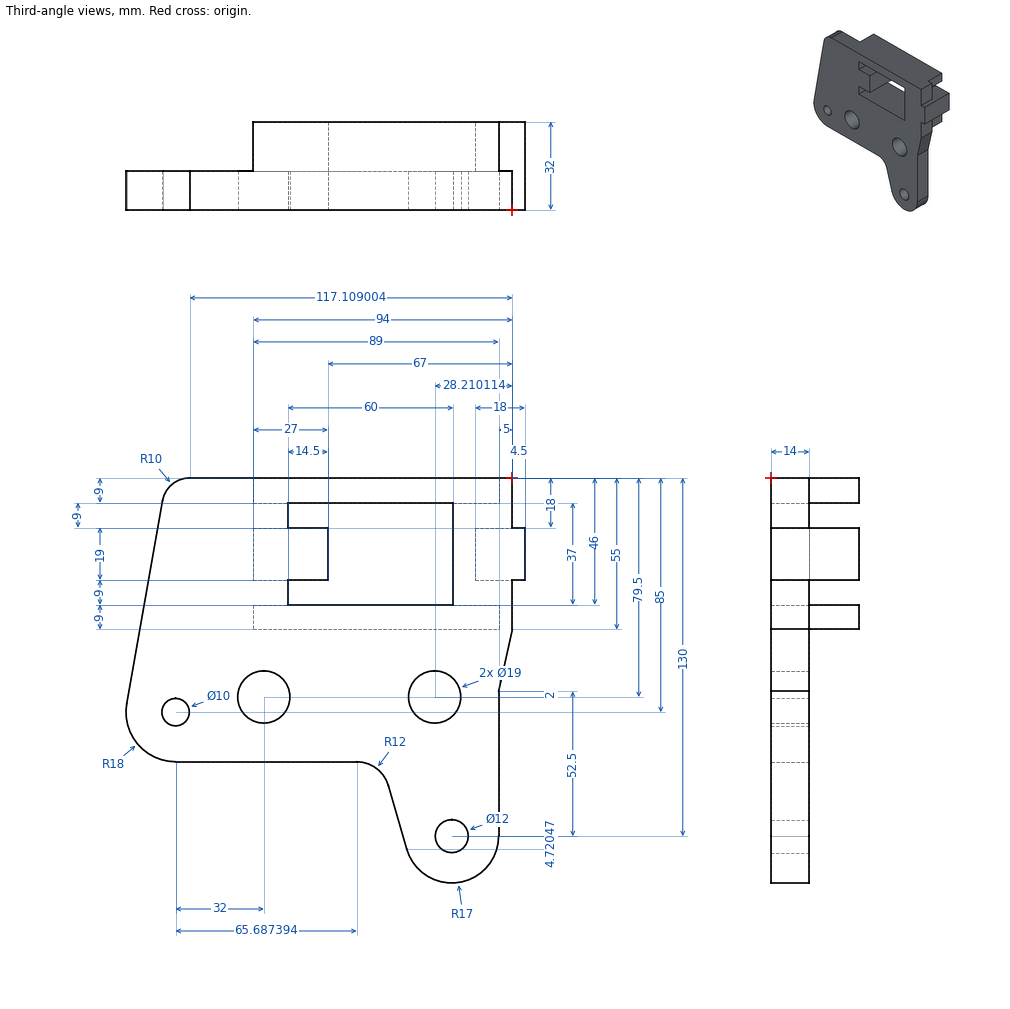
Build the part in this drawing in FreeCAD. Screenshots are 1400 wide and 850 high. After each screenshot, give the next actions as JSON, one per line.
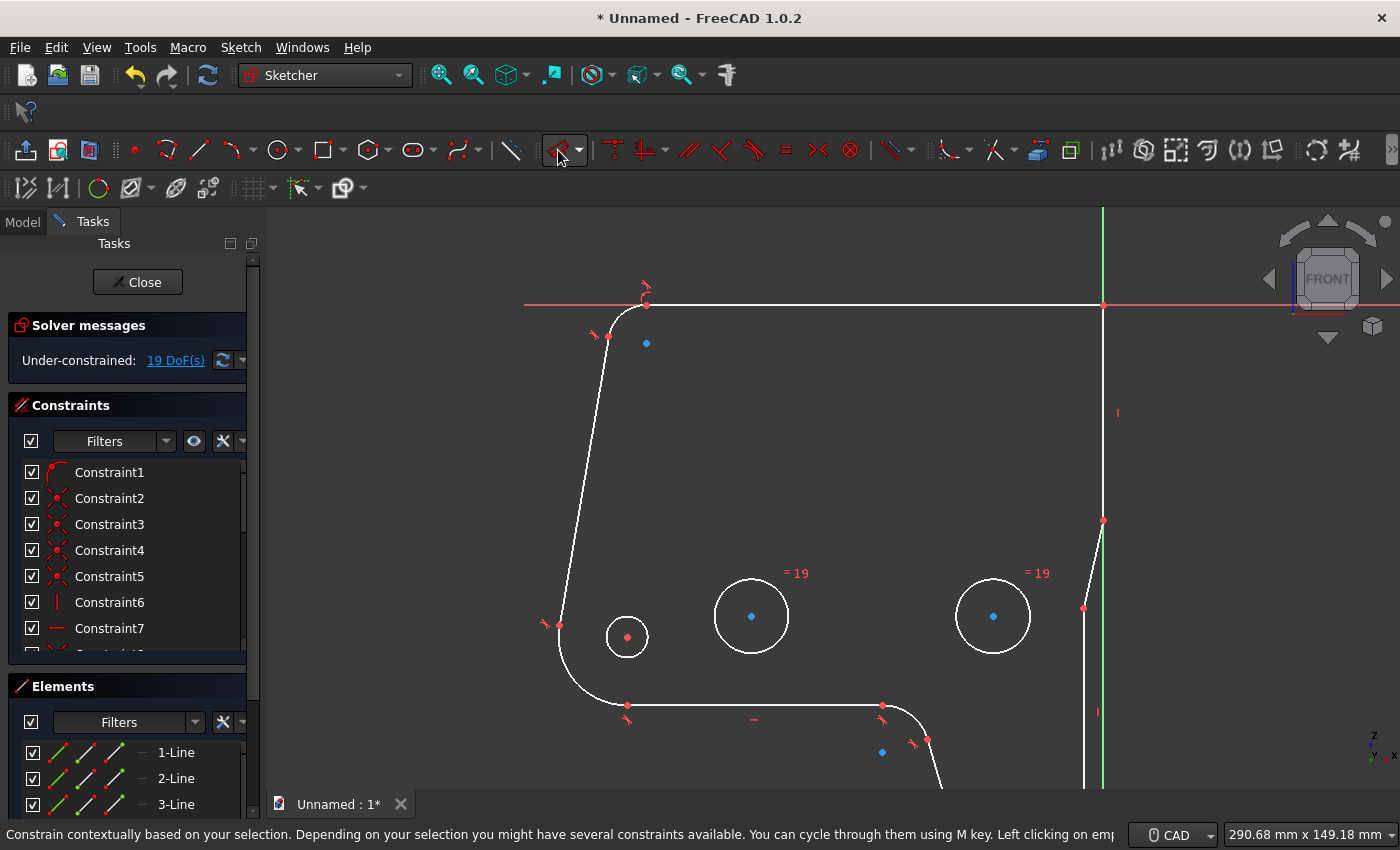
{"action": "scroll", "coordinate": [630, 308], "scroll_direction": "down", "scroll_amount": 2}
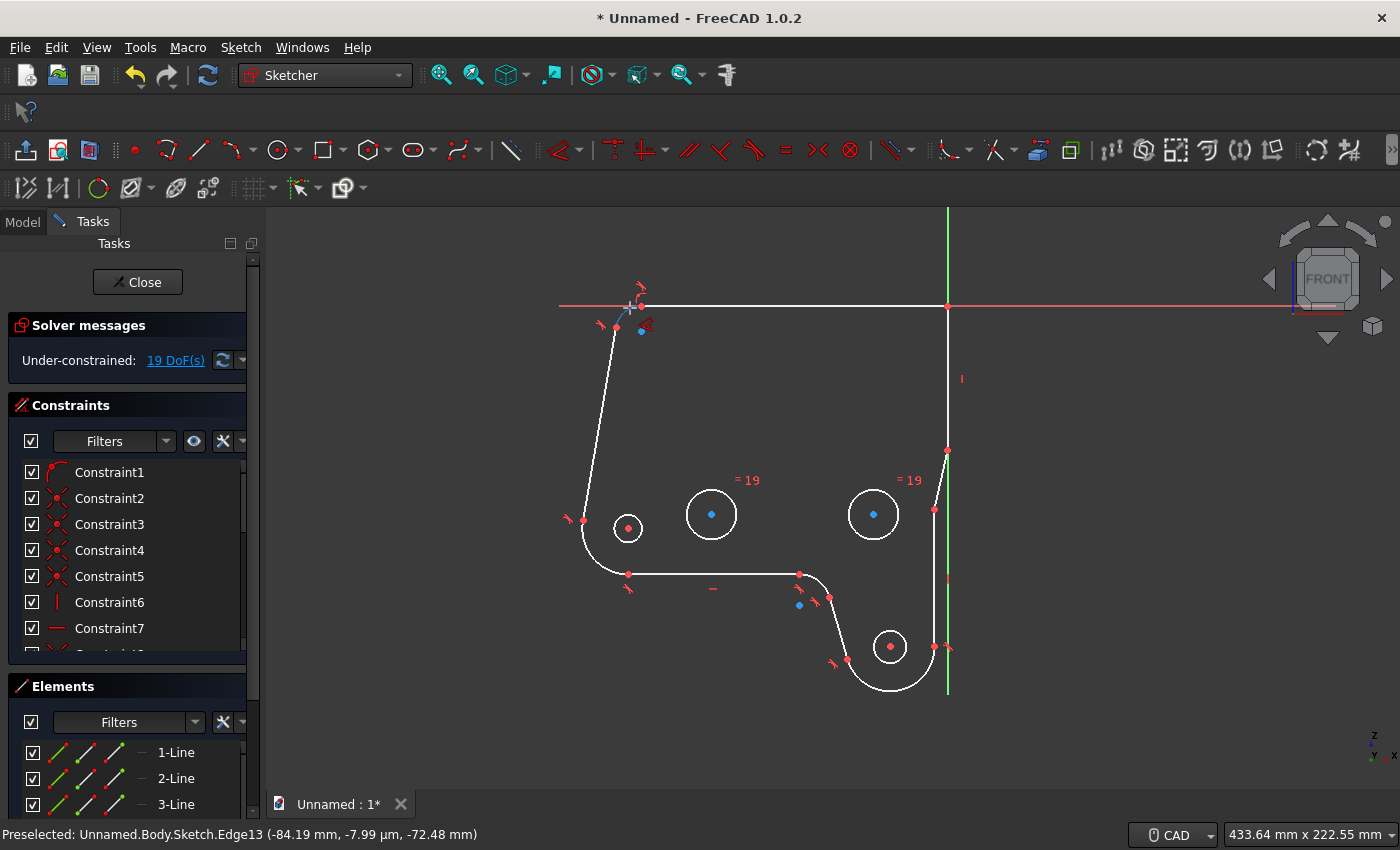
{"action": "left_click", "coordinate": [872, 687]}
{"action": "left_click", "coordinate": [859, 716]}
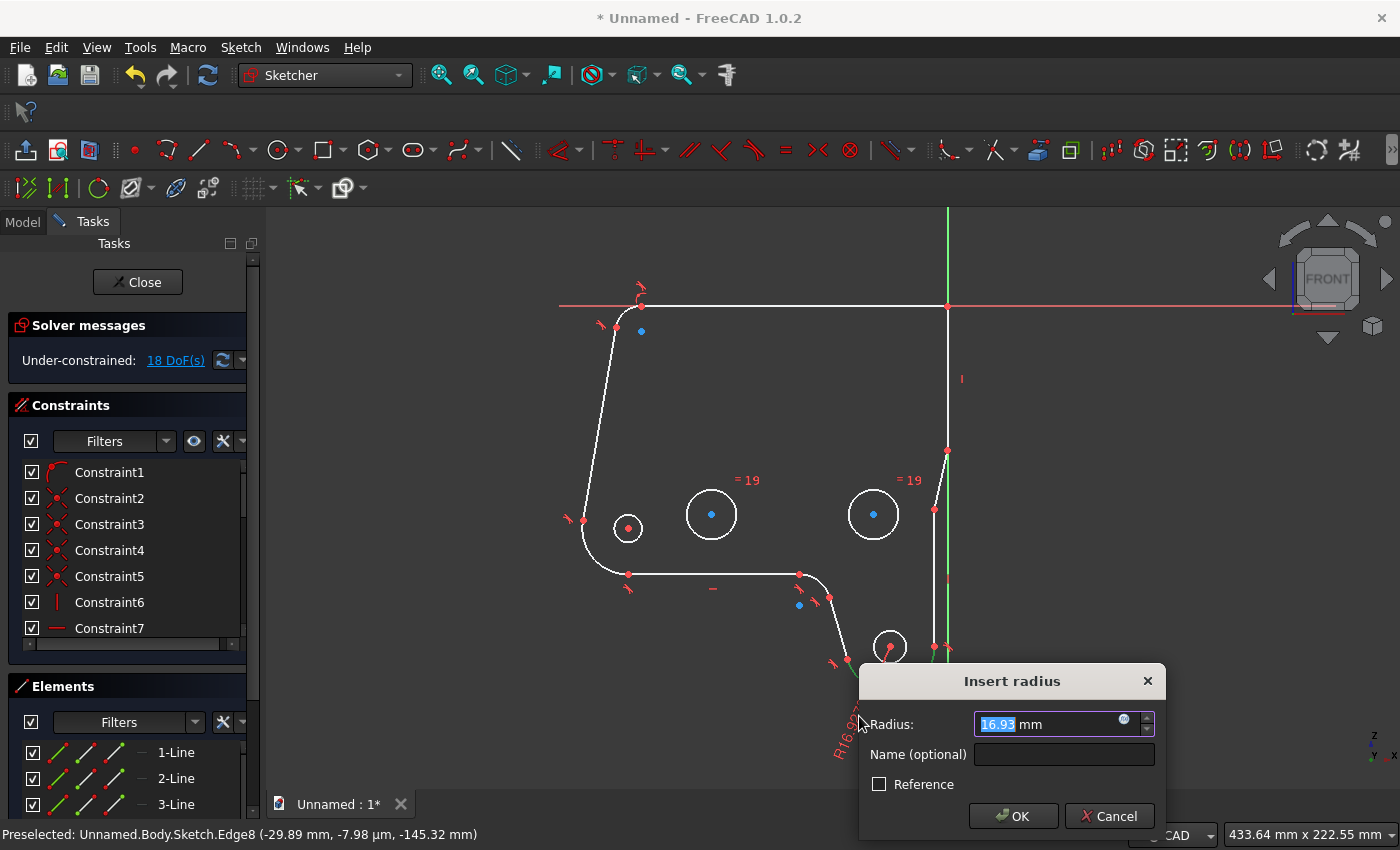
{"action": "type", "text": "17"}
{"action": "key", "text": "Return"}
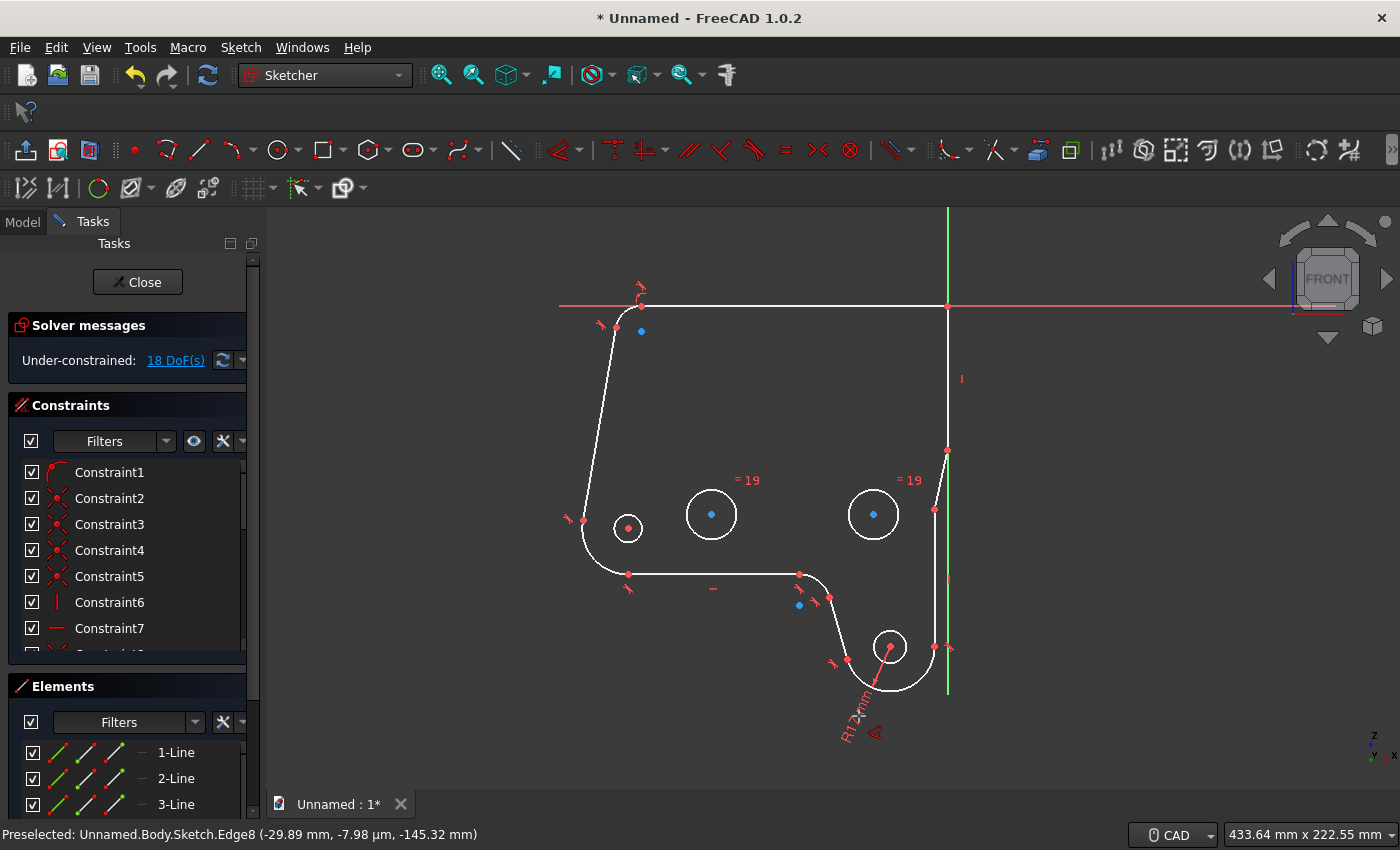
{"action": "scroll", "coordinate": [824, 586], "scroll_direction": "up", "scroll_amount": 2}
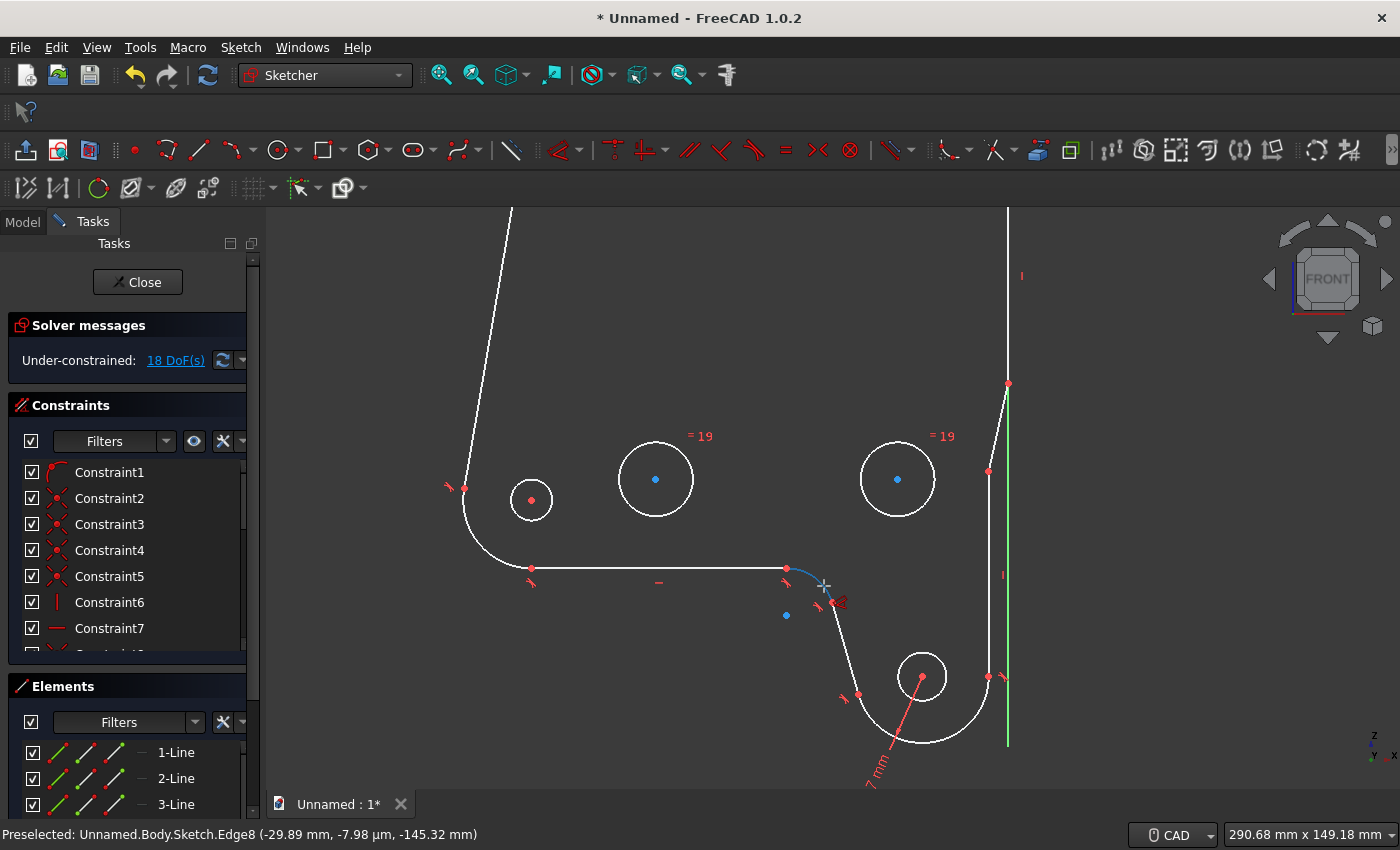
{"action": "left_click", "coordinate": [824, 586]}
{"action": "left_click", "coordinate": [849, 566]}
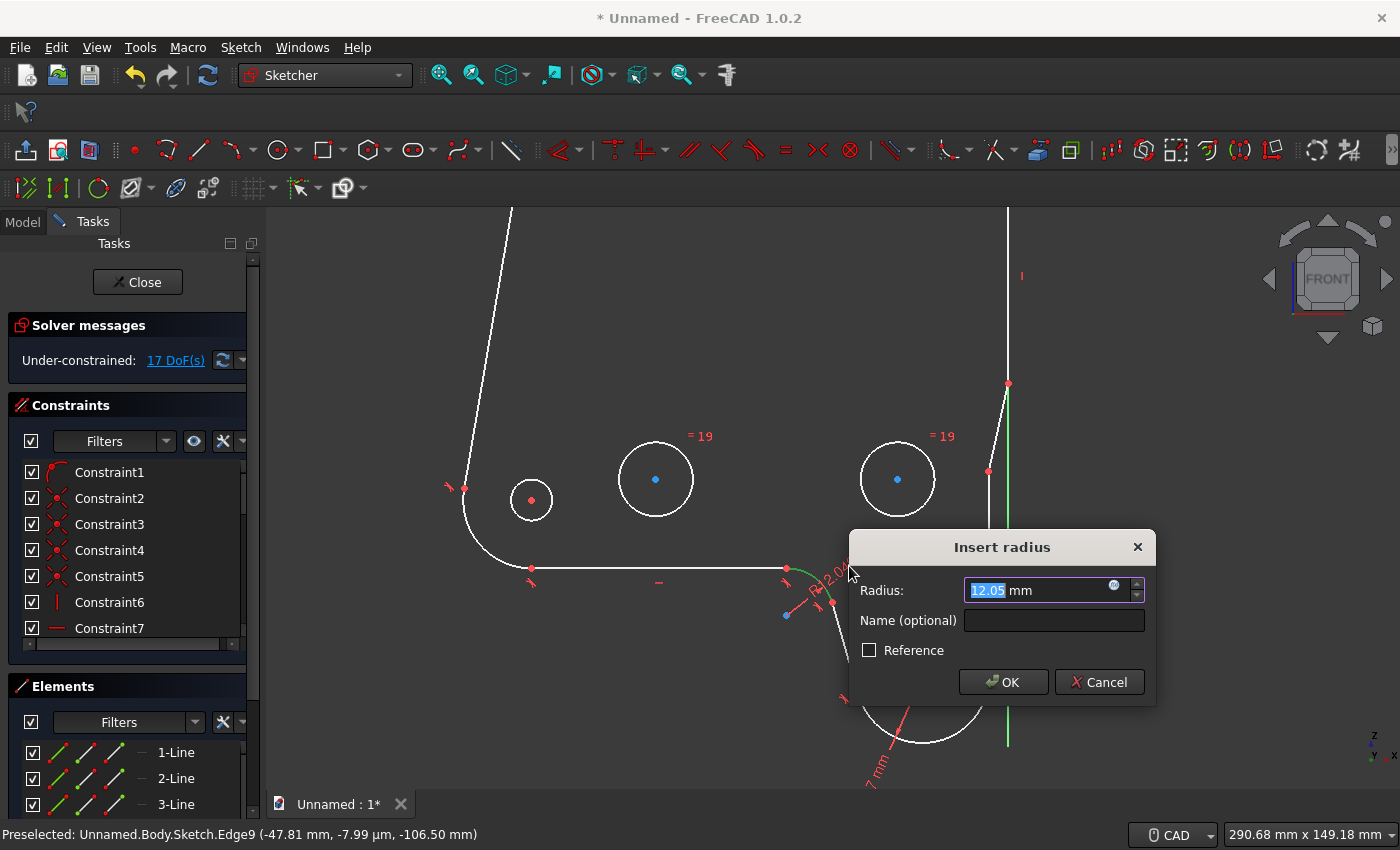
{"action": "type", "text": "12"}
{"action": "key", "text": "Return"}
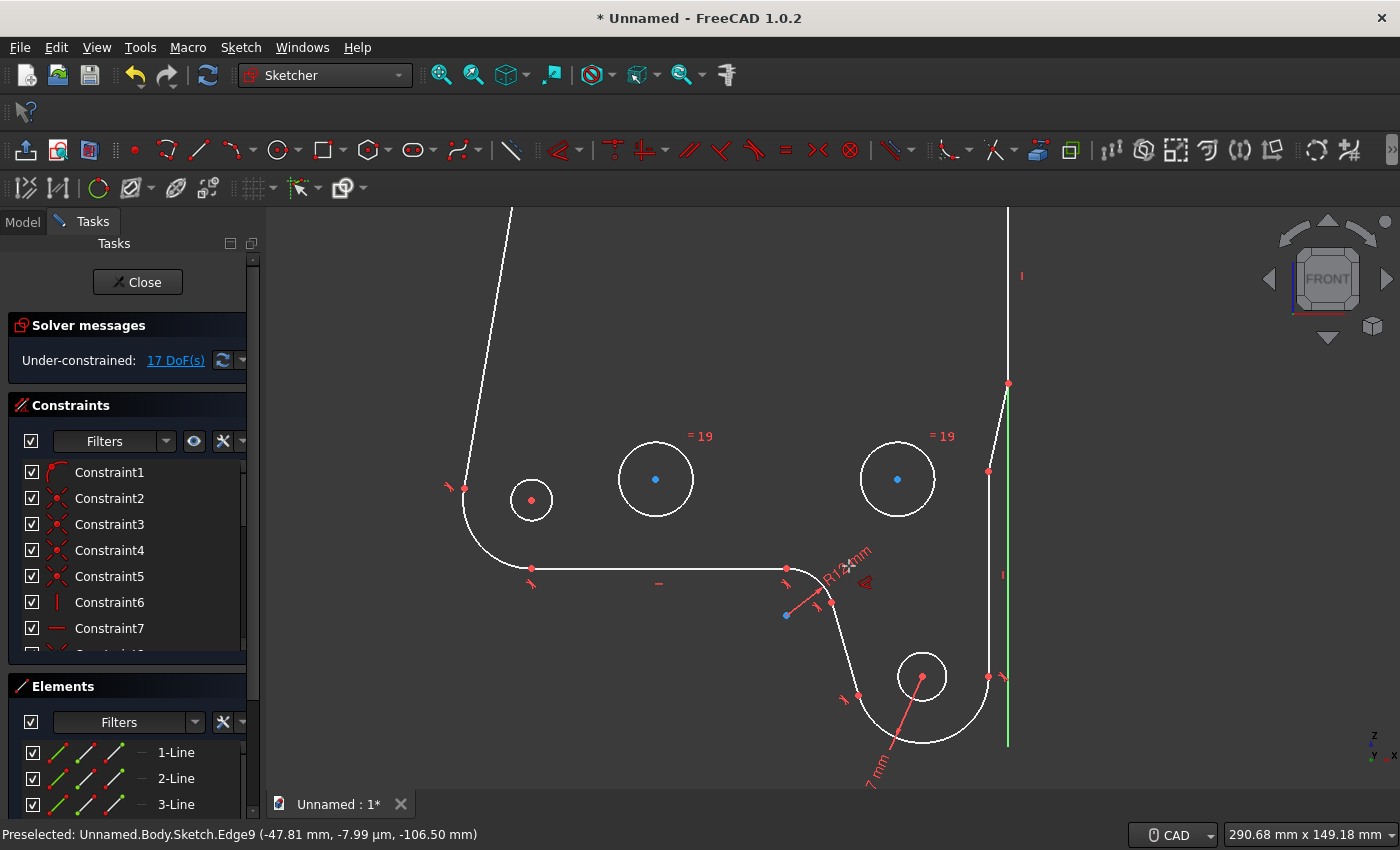
{"action": "left_click", "coordinate": [467, 524]}
{"action": "left_click", "coordinate": [437, 535]}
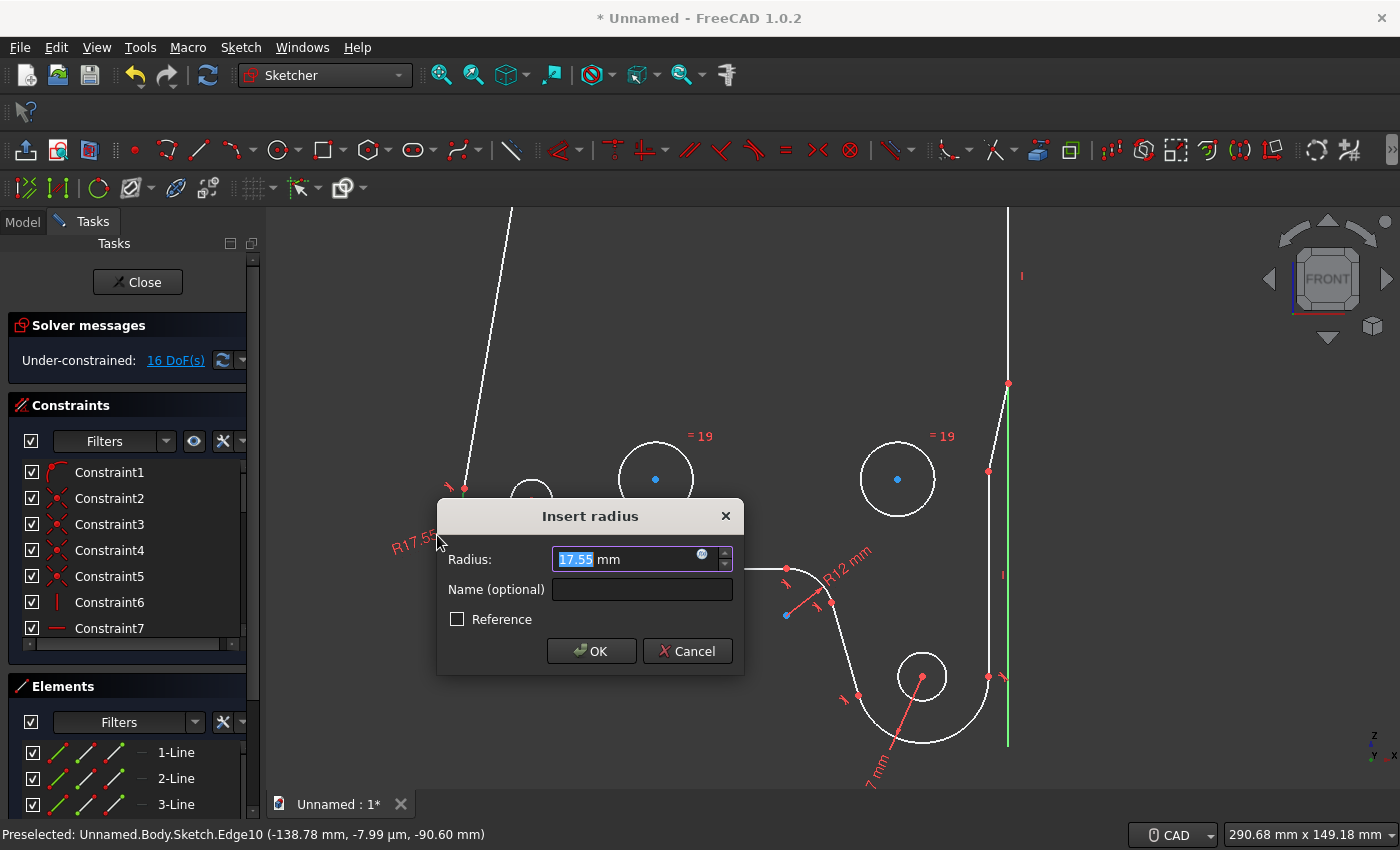
{"action": "type", "text": "18"}
{"action": "key", "text": "Return"}